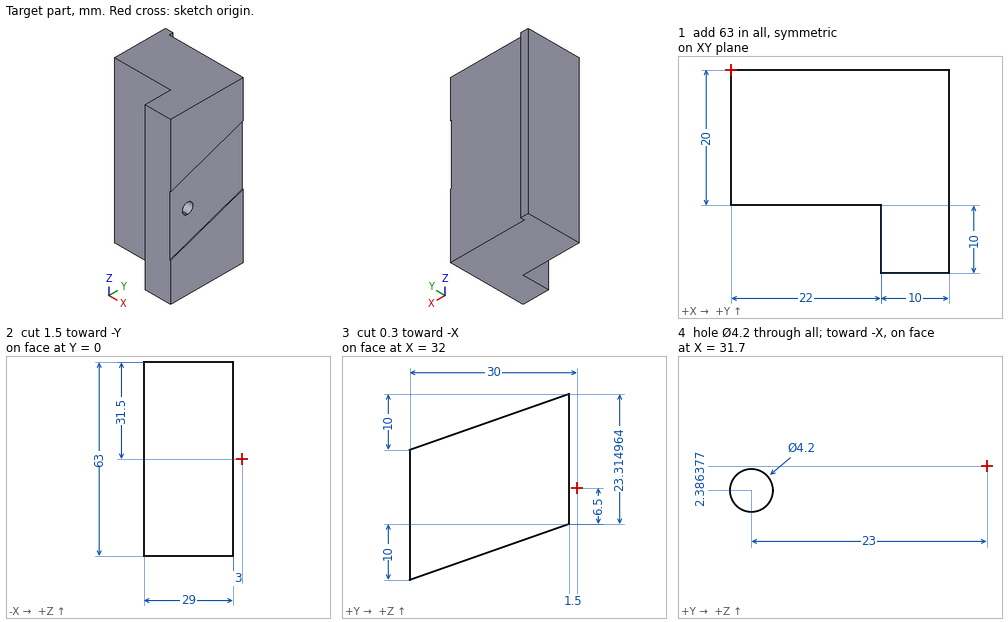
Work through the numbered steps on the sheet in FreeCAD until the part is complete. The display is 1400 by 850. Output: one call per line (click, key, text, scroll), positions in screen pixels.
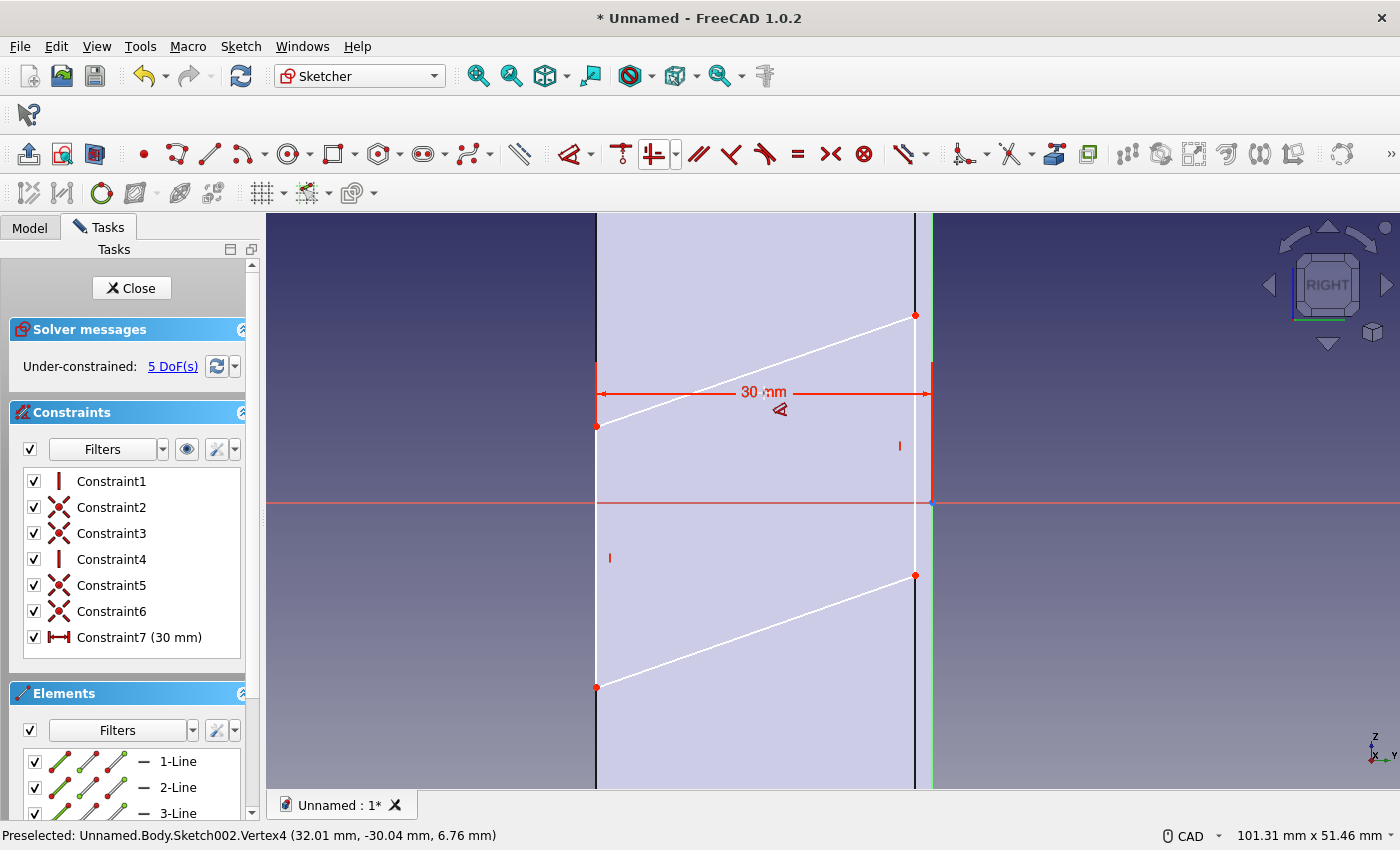
click(819, 349)
click(562, 371)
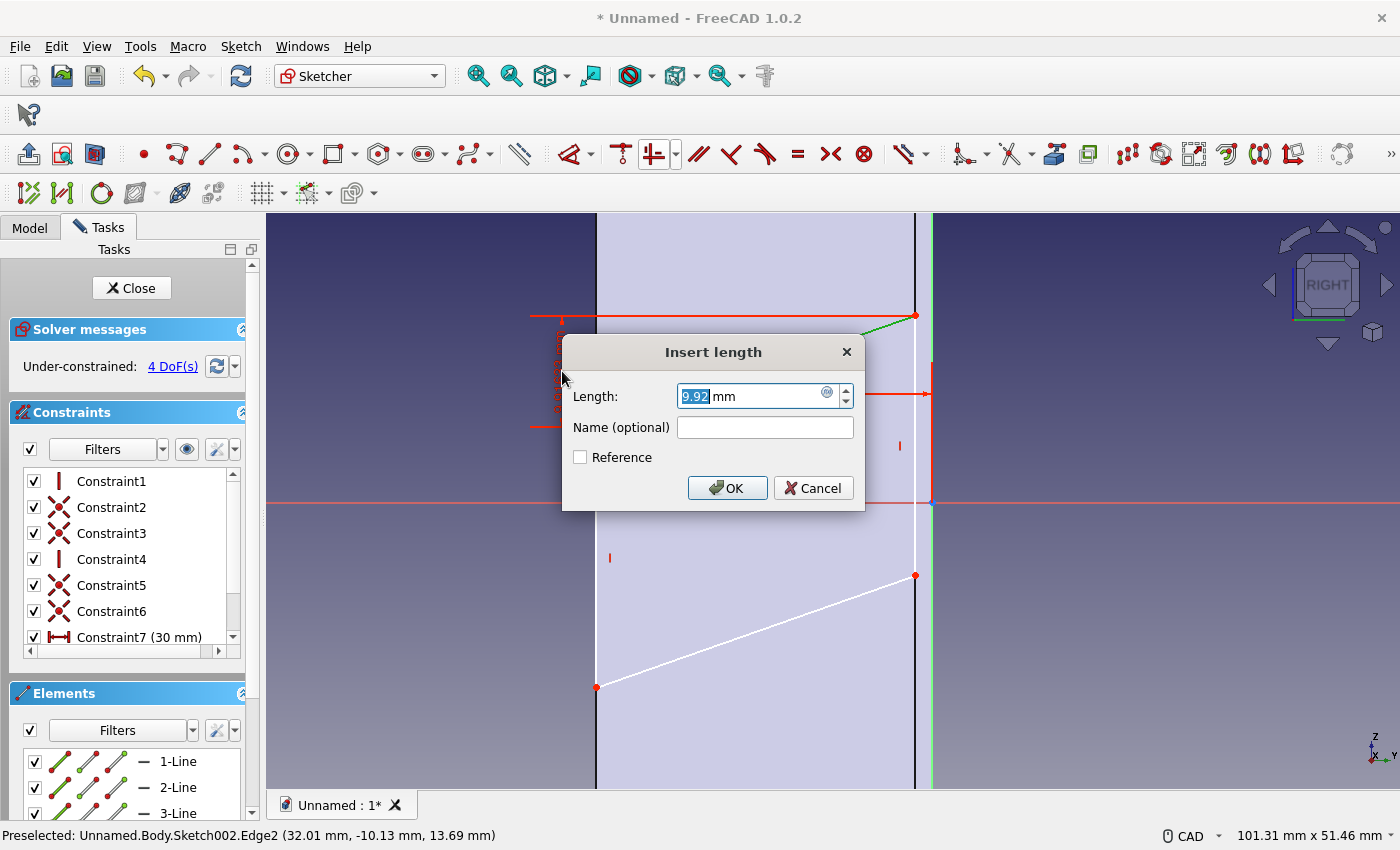
text(10)
key(Return)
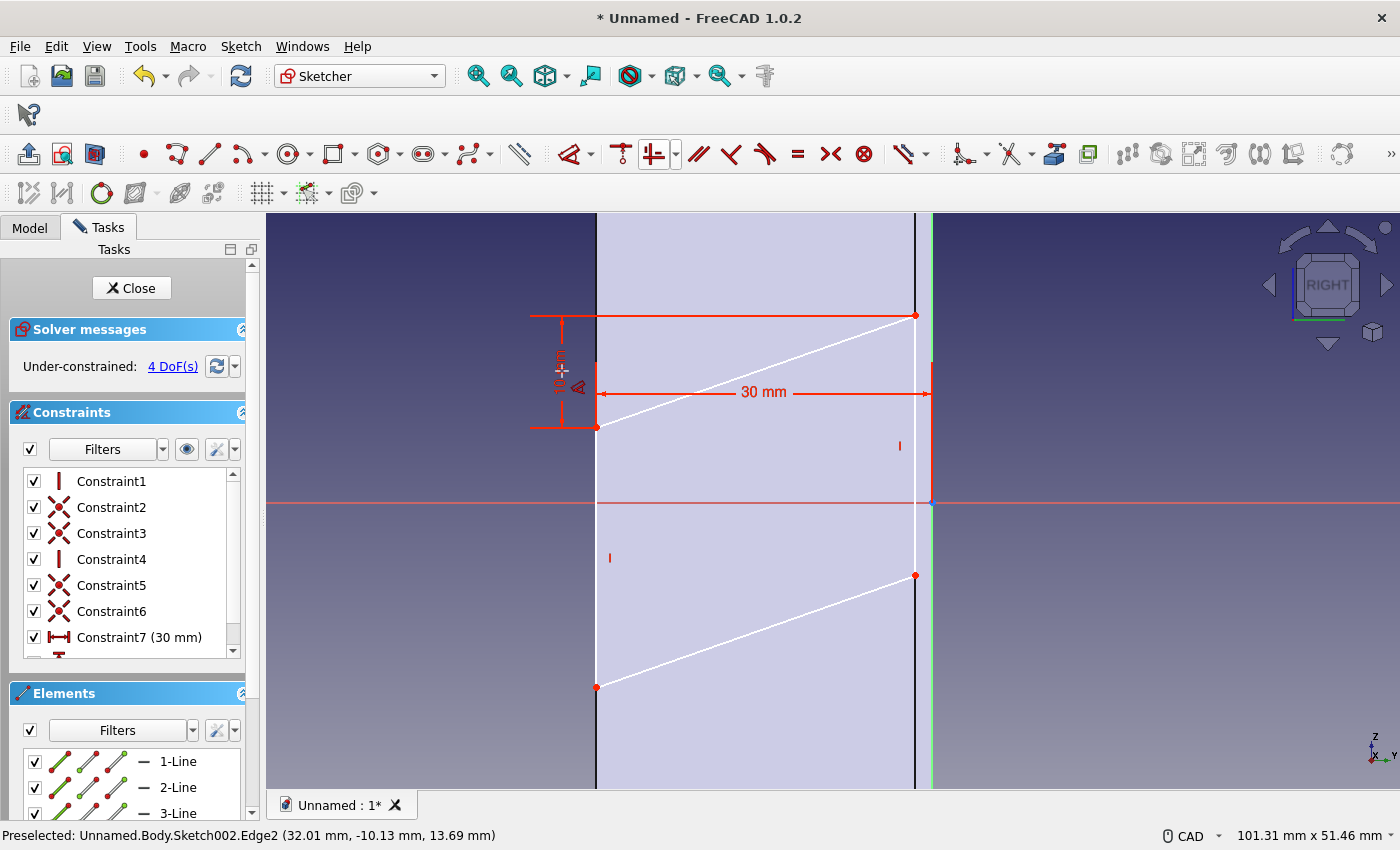
click(692, 654)
click(562, 632)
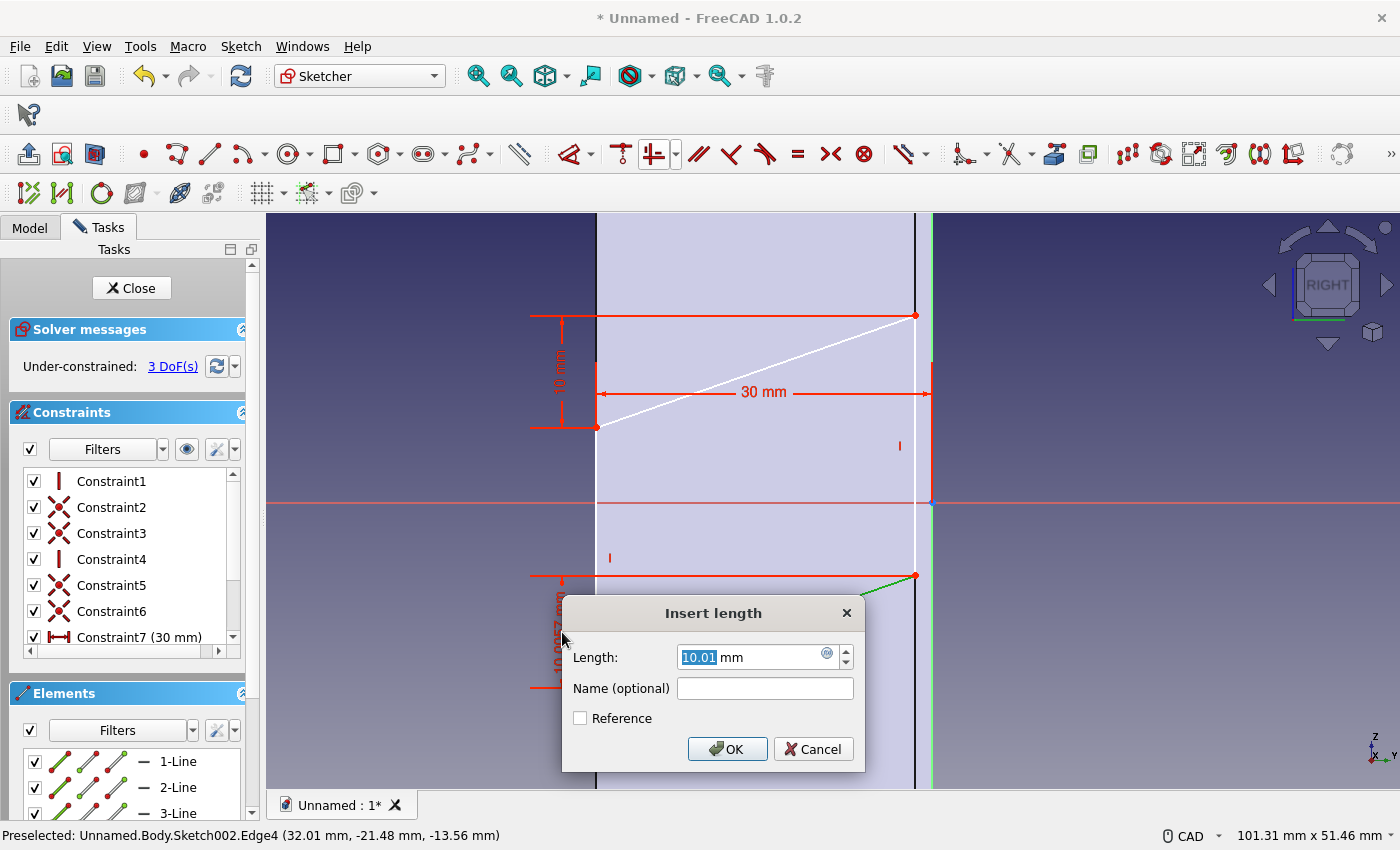
text(10)
key(Return)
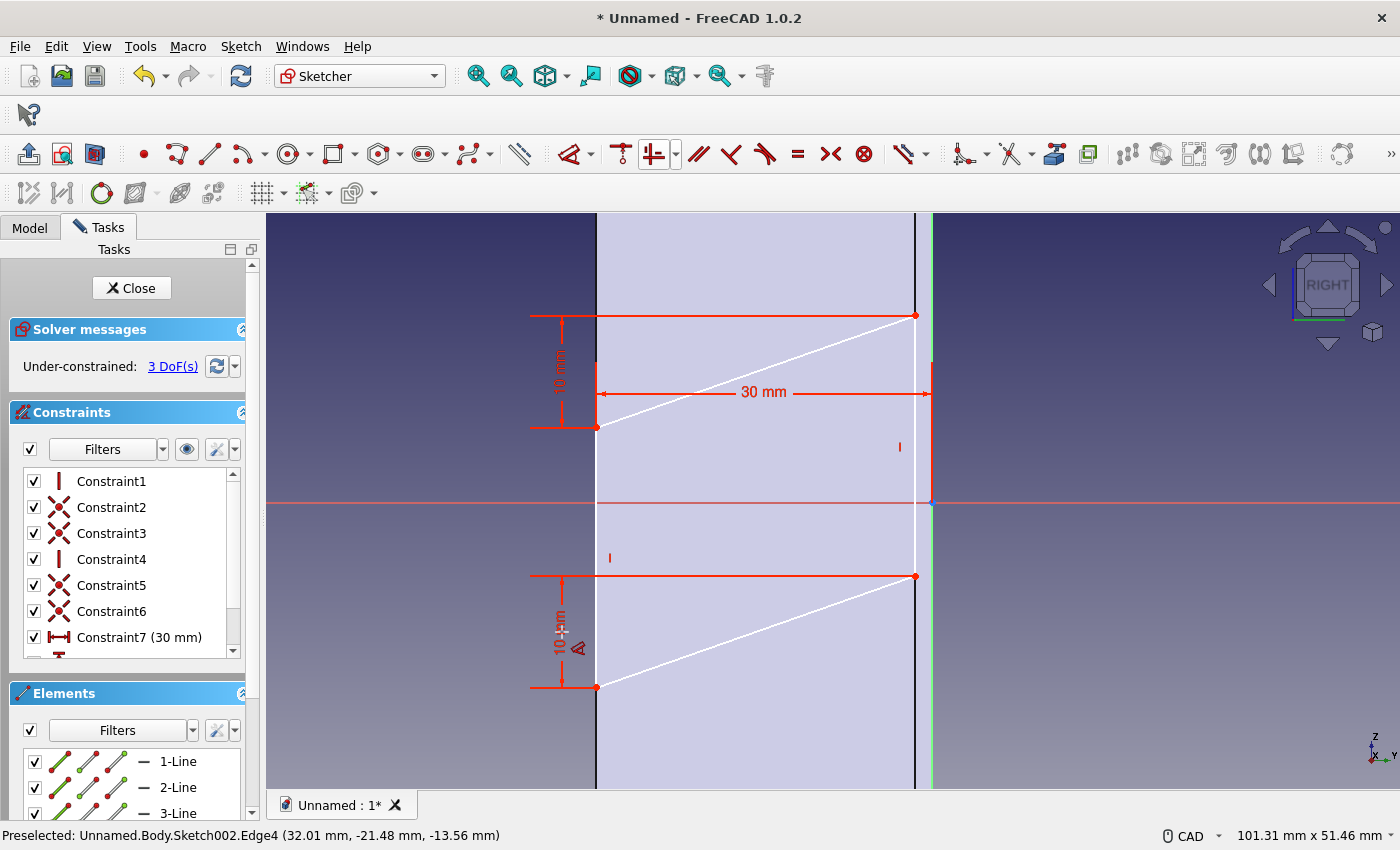
scroll(915, 576, up, 5)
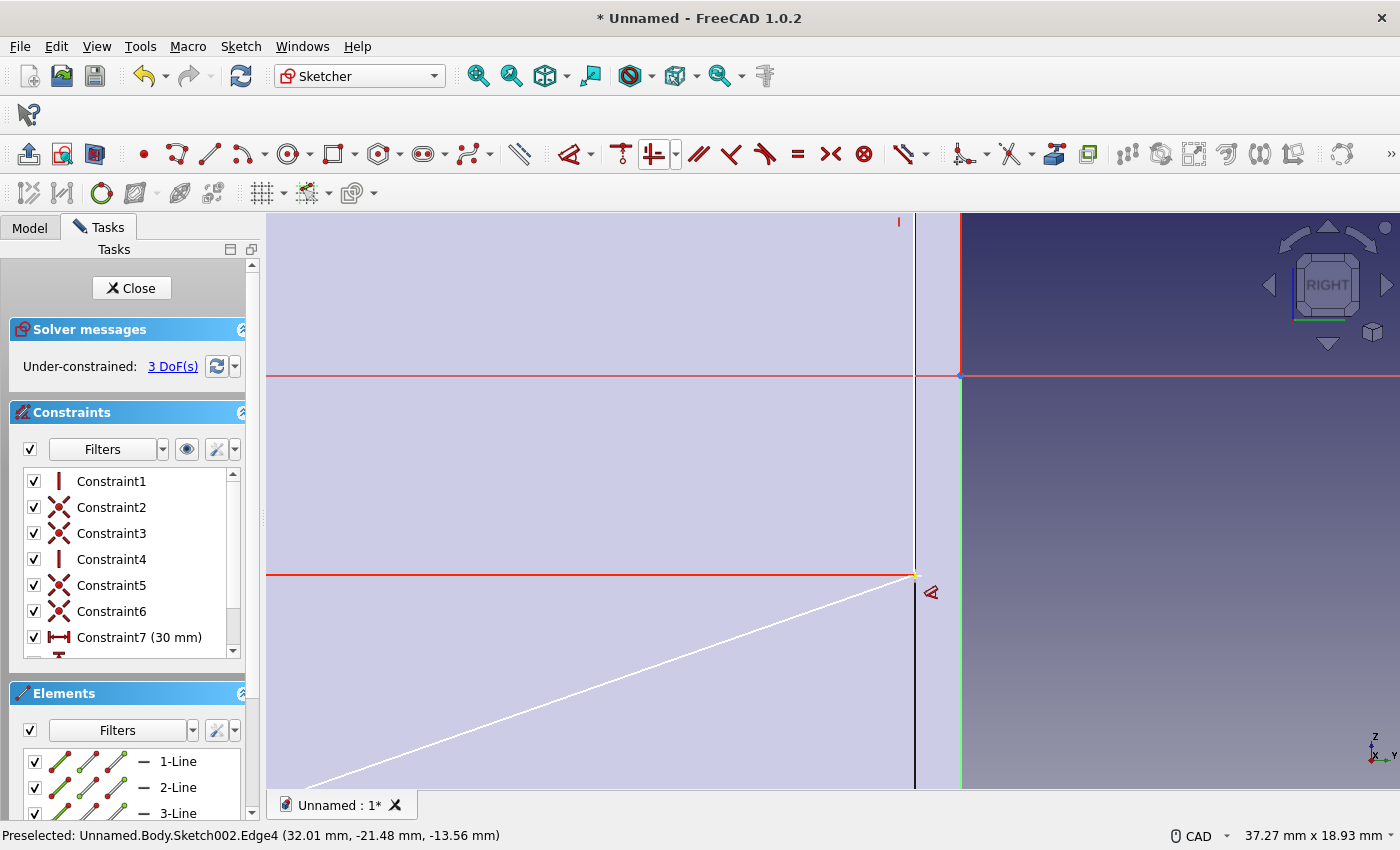
click(914, 575)
click(937, 609)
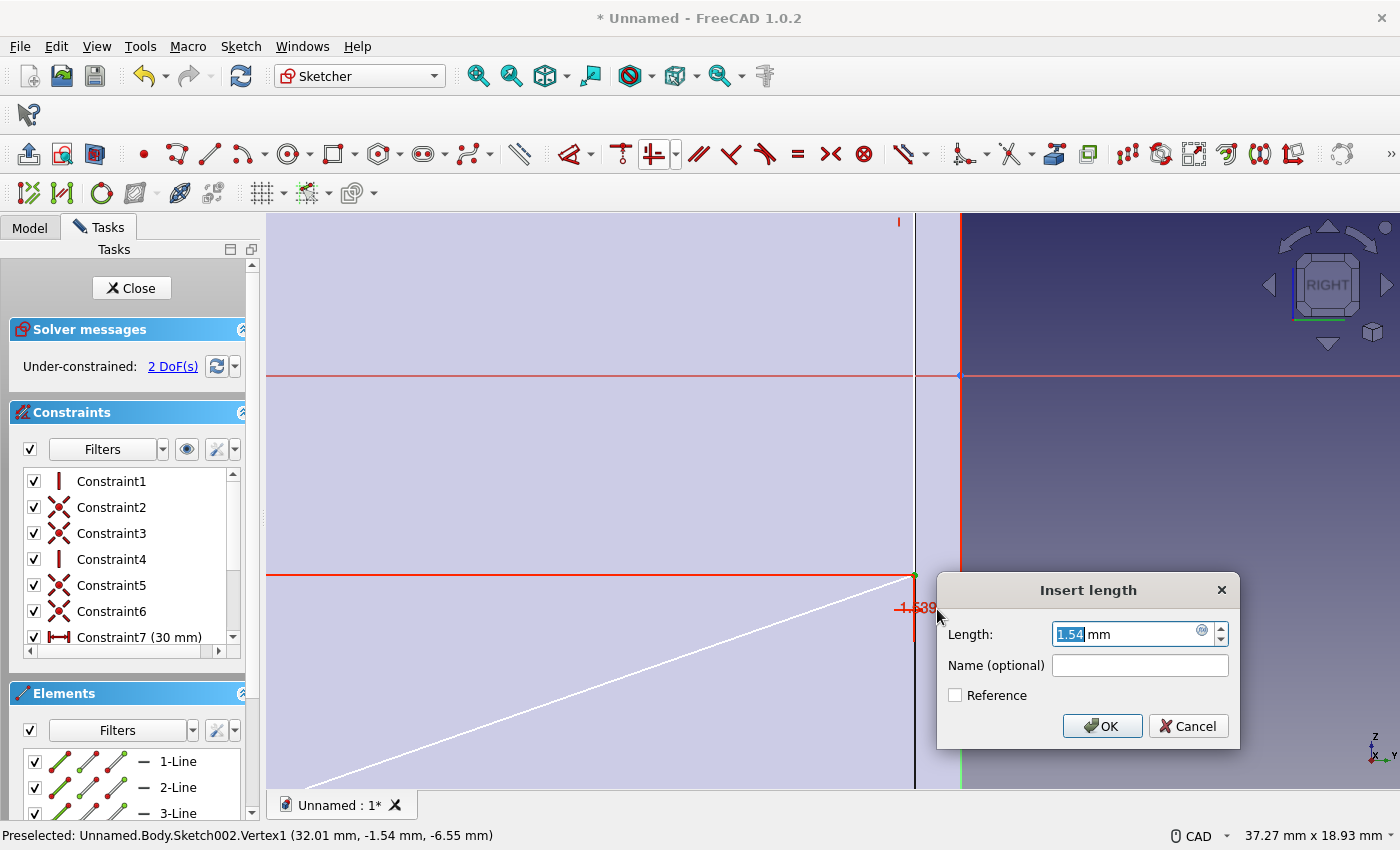
text(1.5)
key(Return)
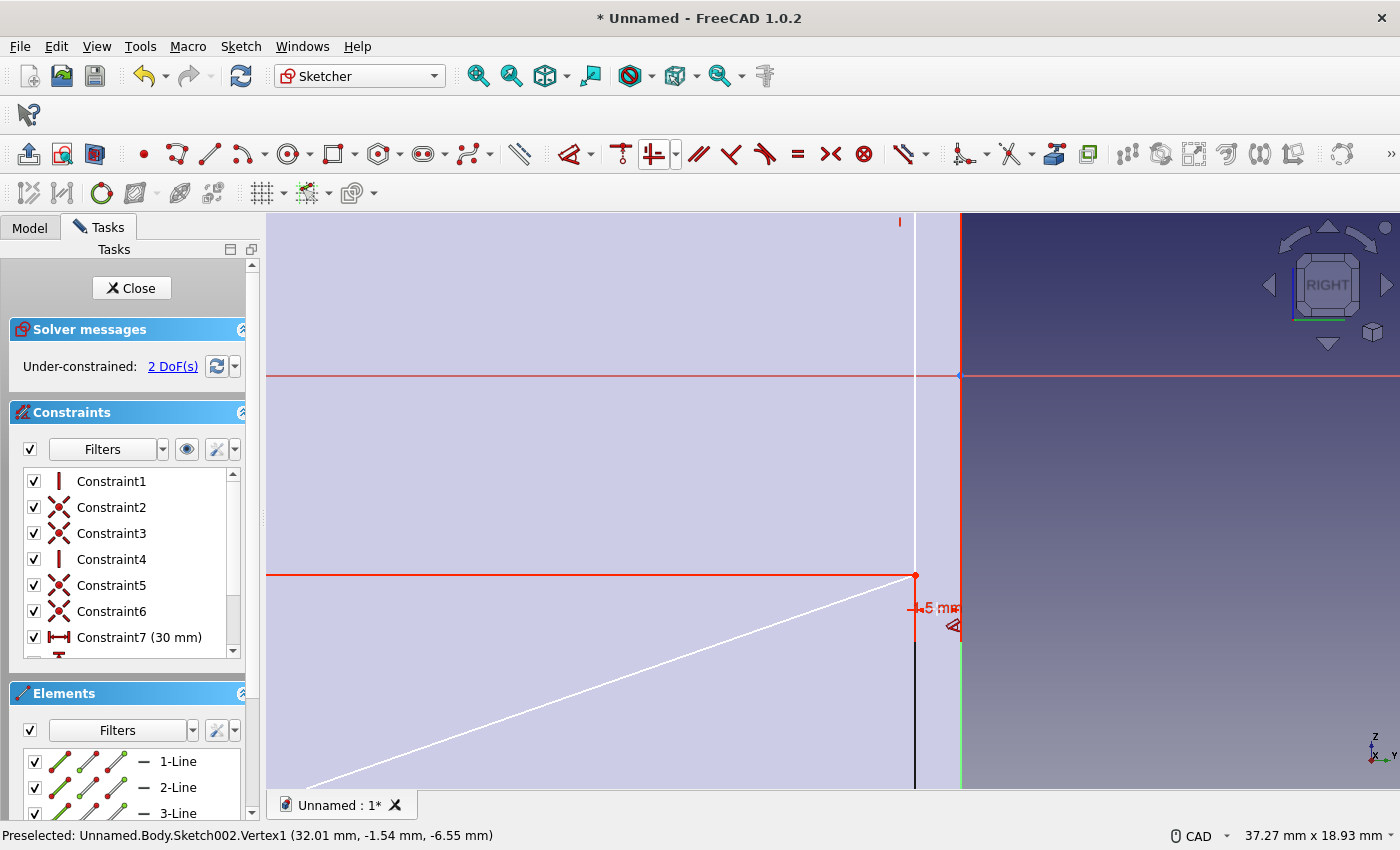
click(915, 575)
click(995, 475)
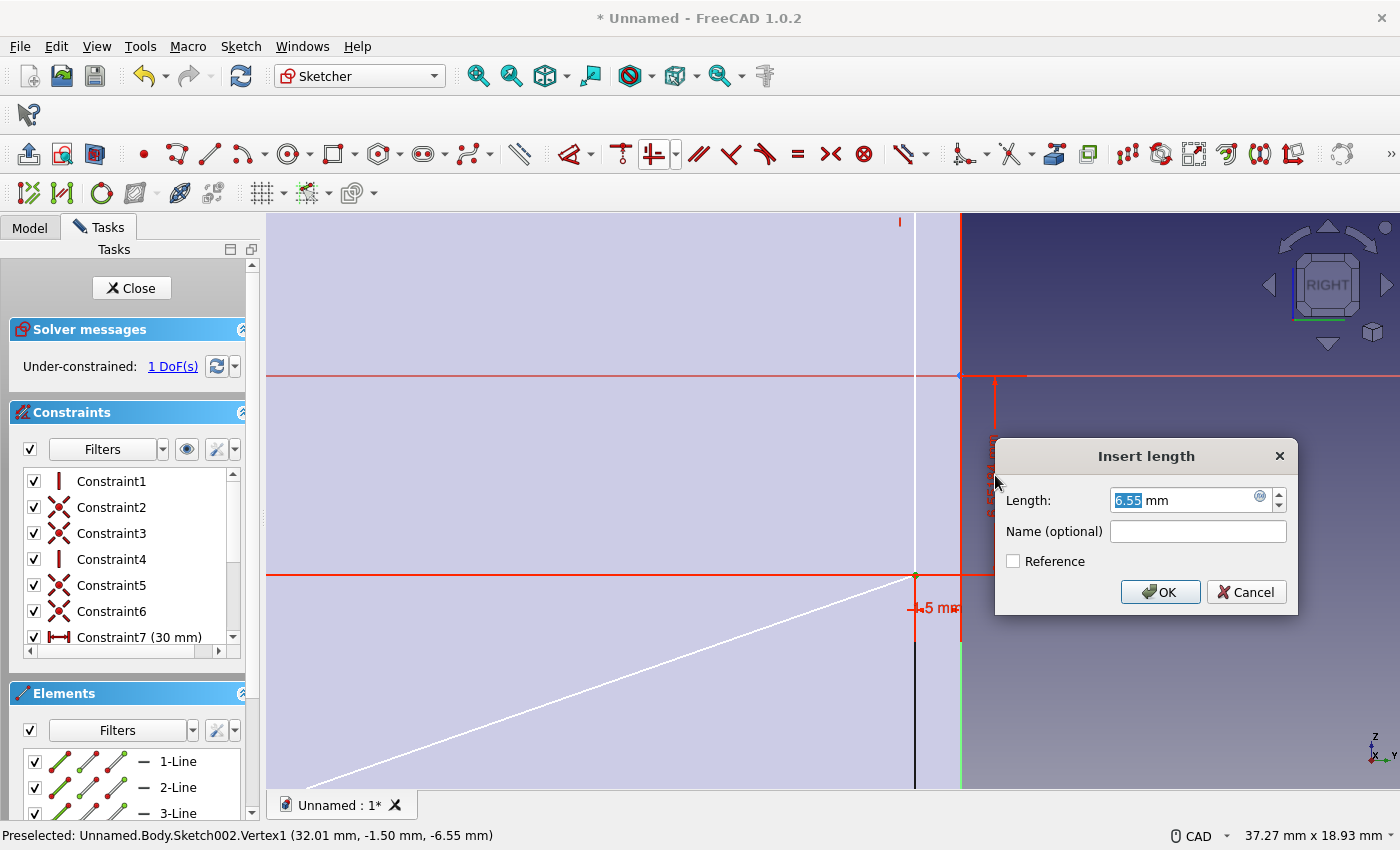
text(6.5)
key(Return)